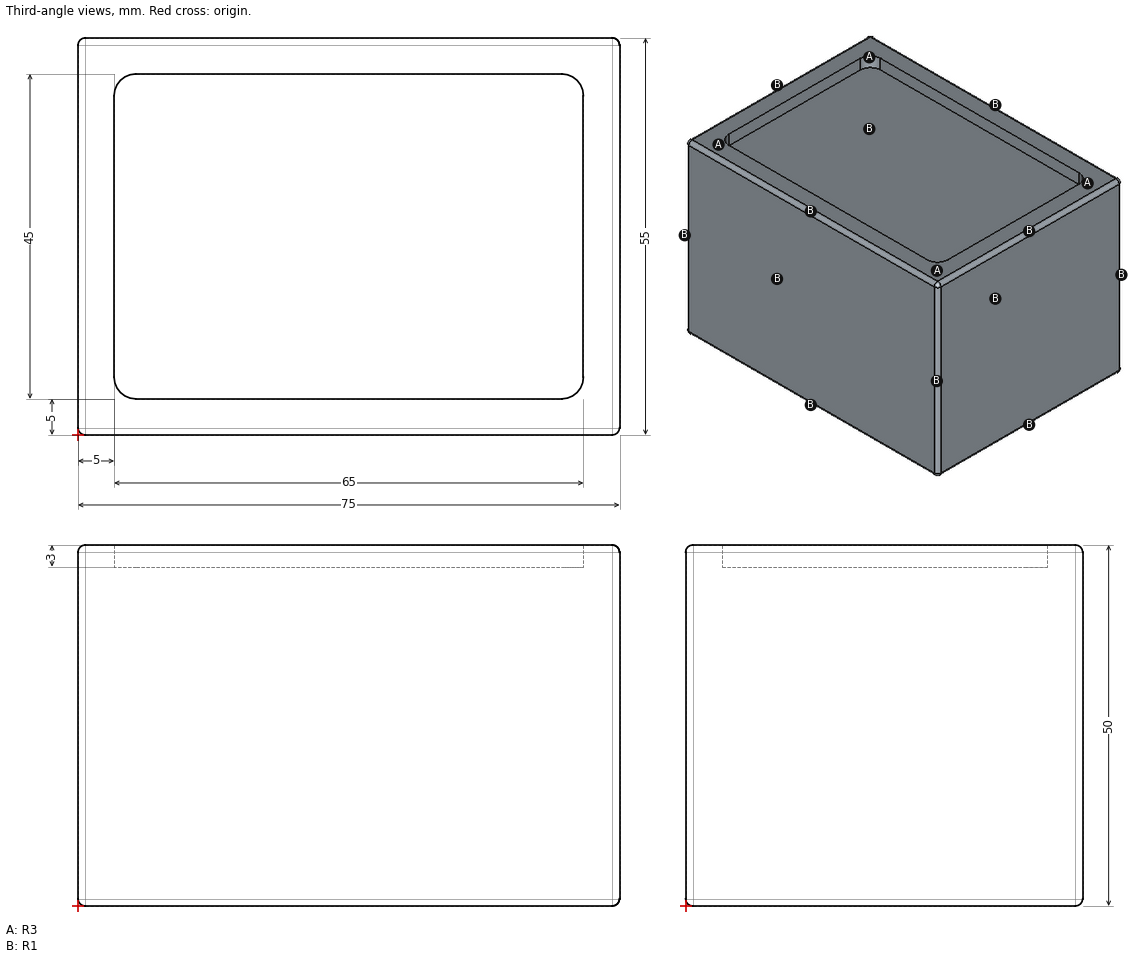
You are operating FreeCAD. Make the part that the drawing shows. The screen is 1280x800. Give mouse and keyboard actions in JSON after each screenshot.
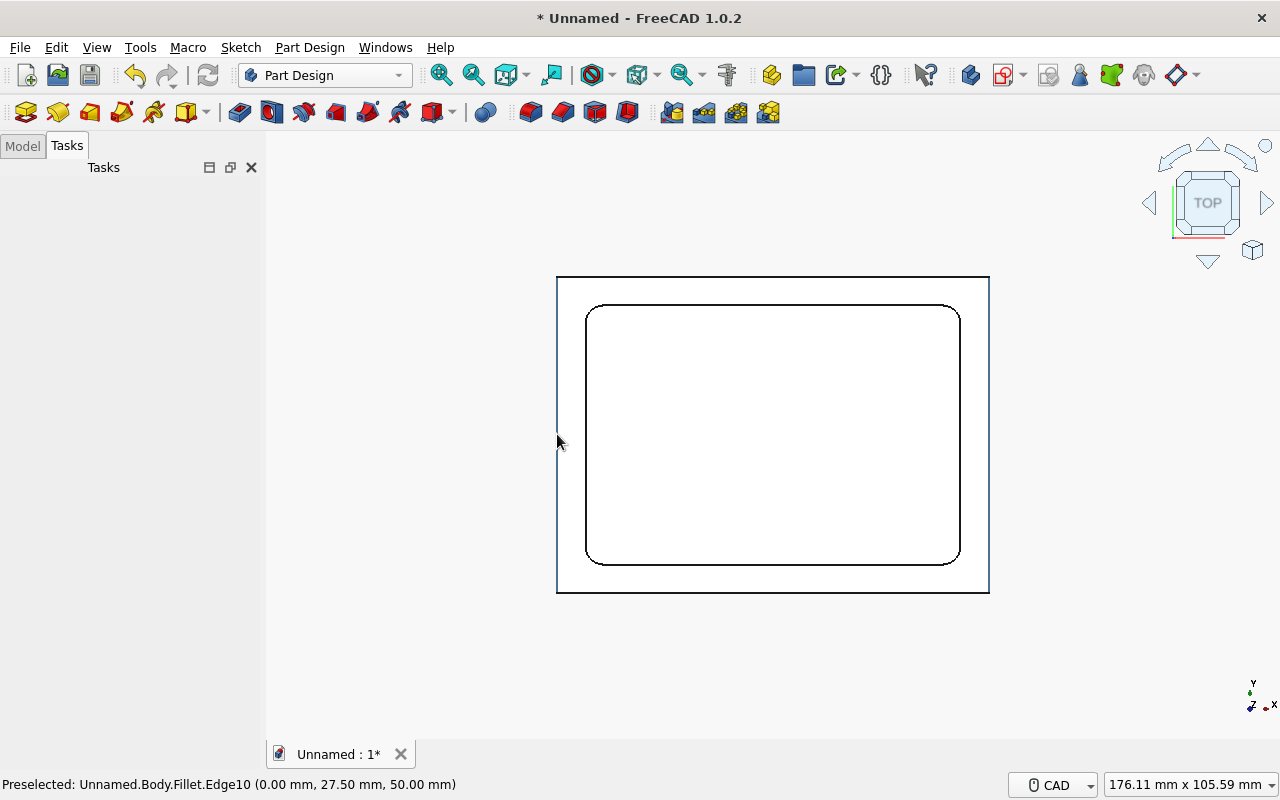
{"action": "key", "text": "0"}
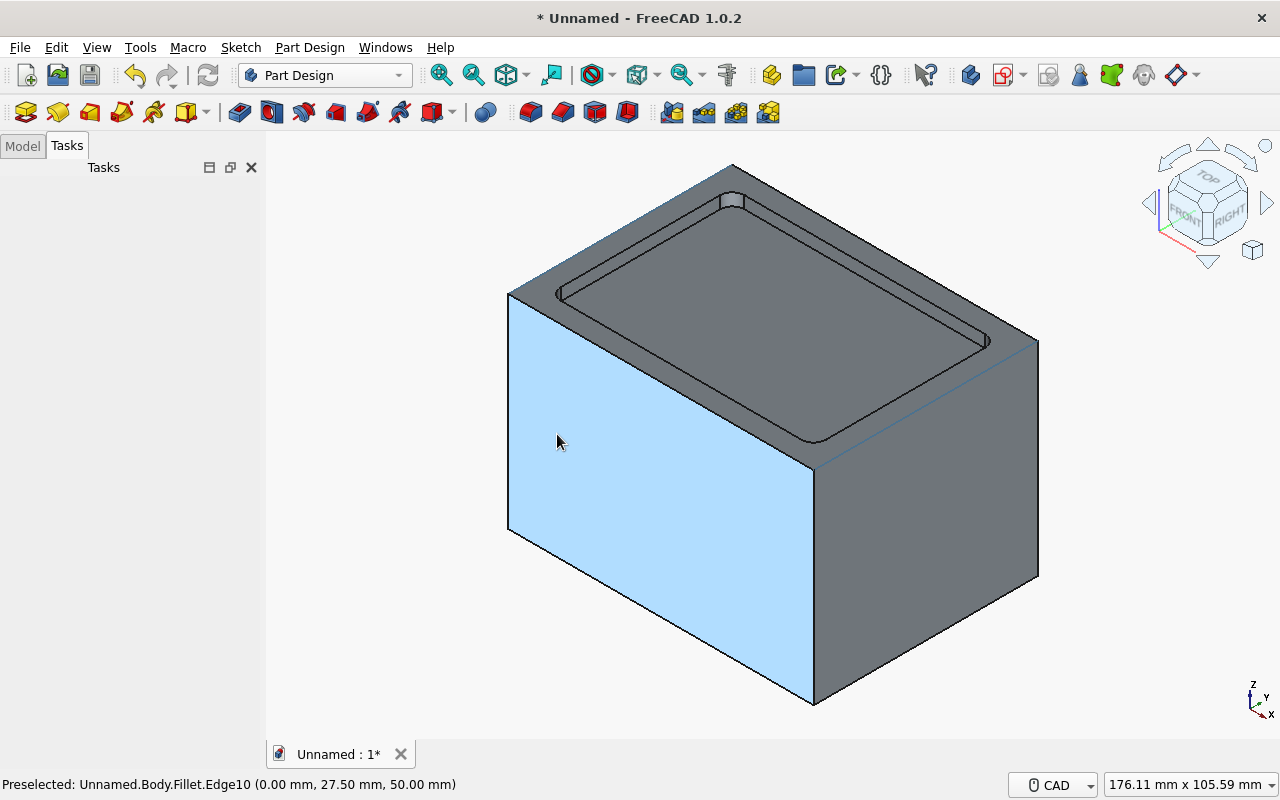
{"action": "key", "text": "1"}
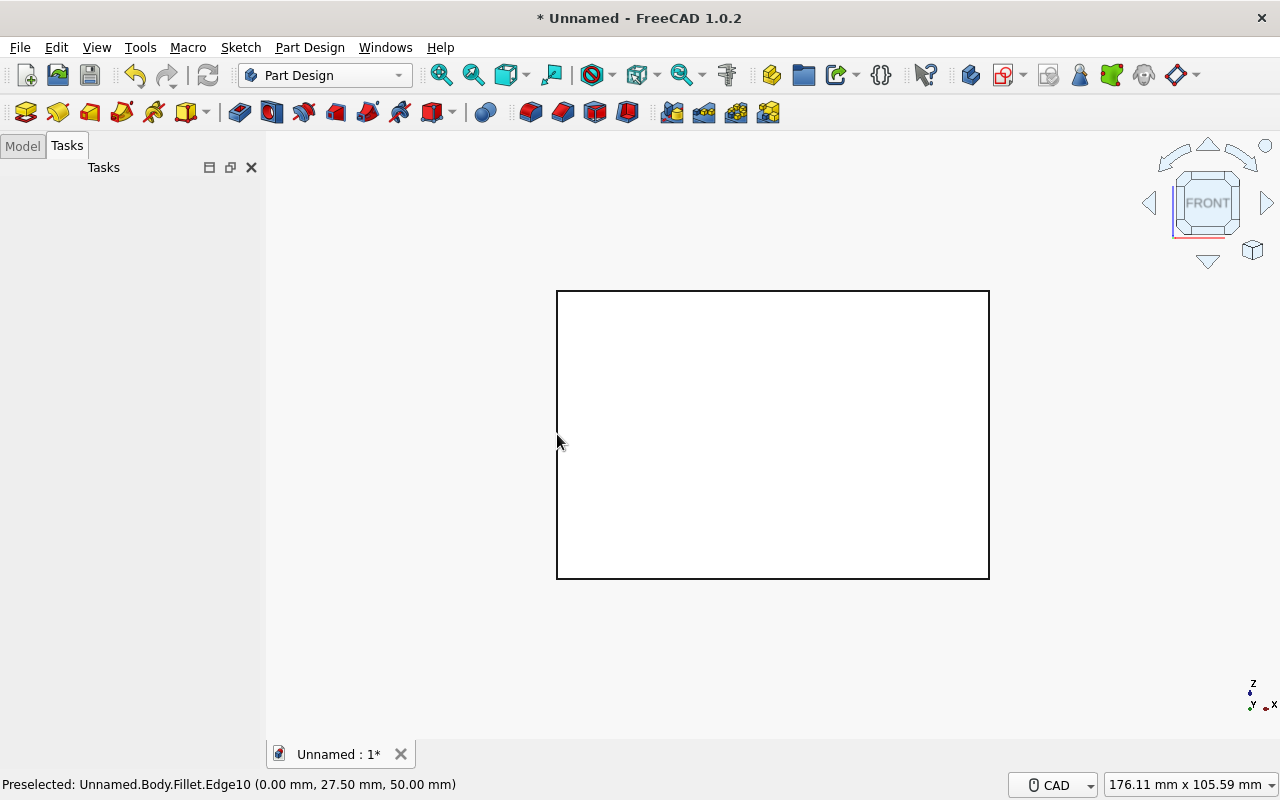
{"action": "key", "text": "3"}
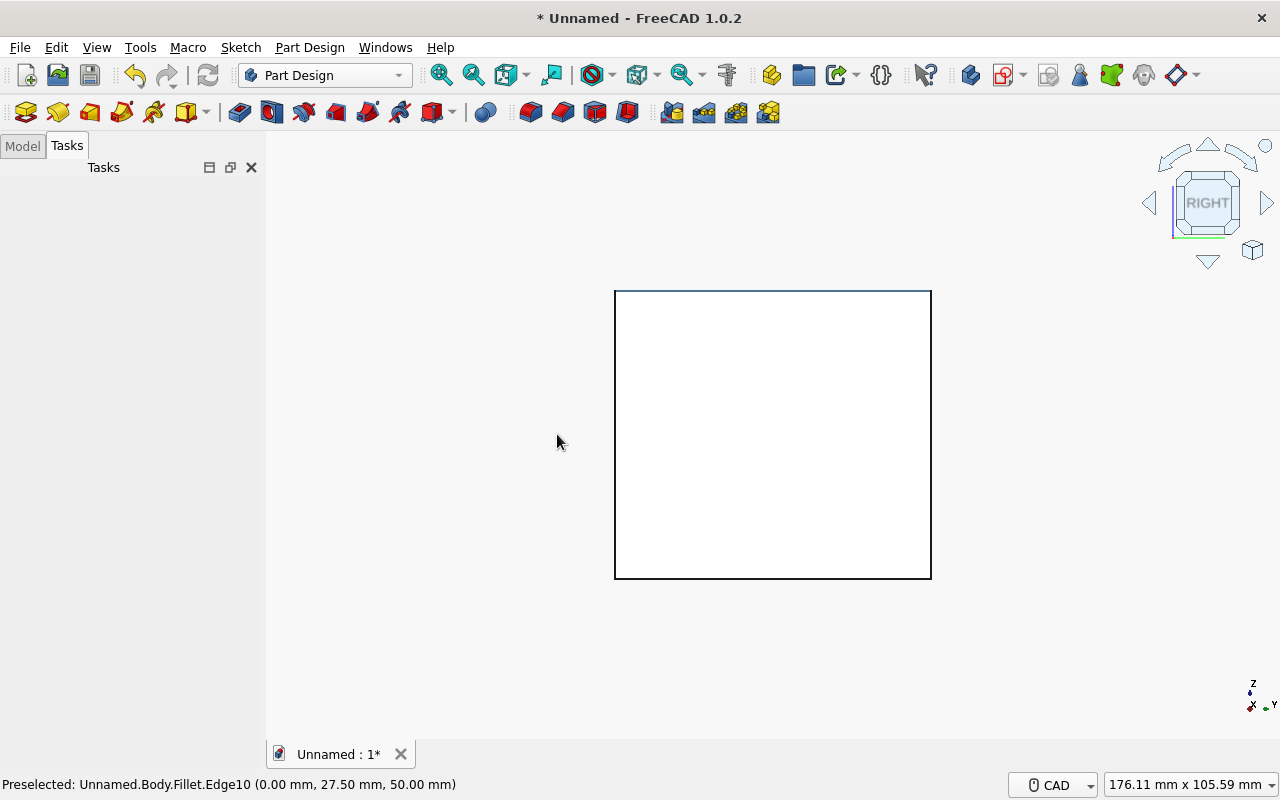
{"action": "key", "text": "5"}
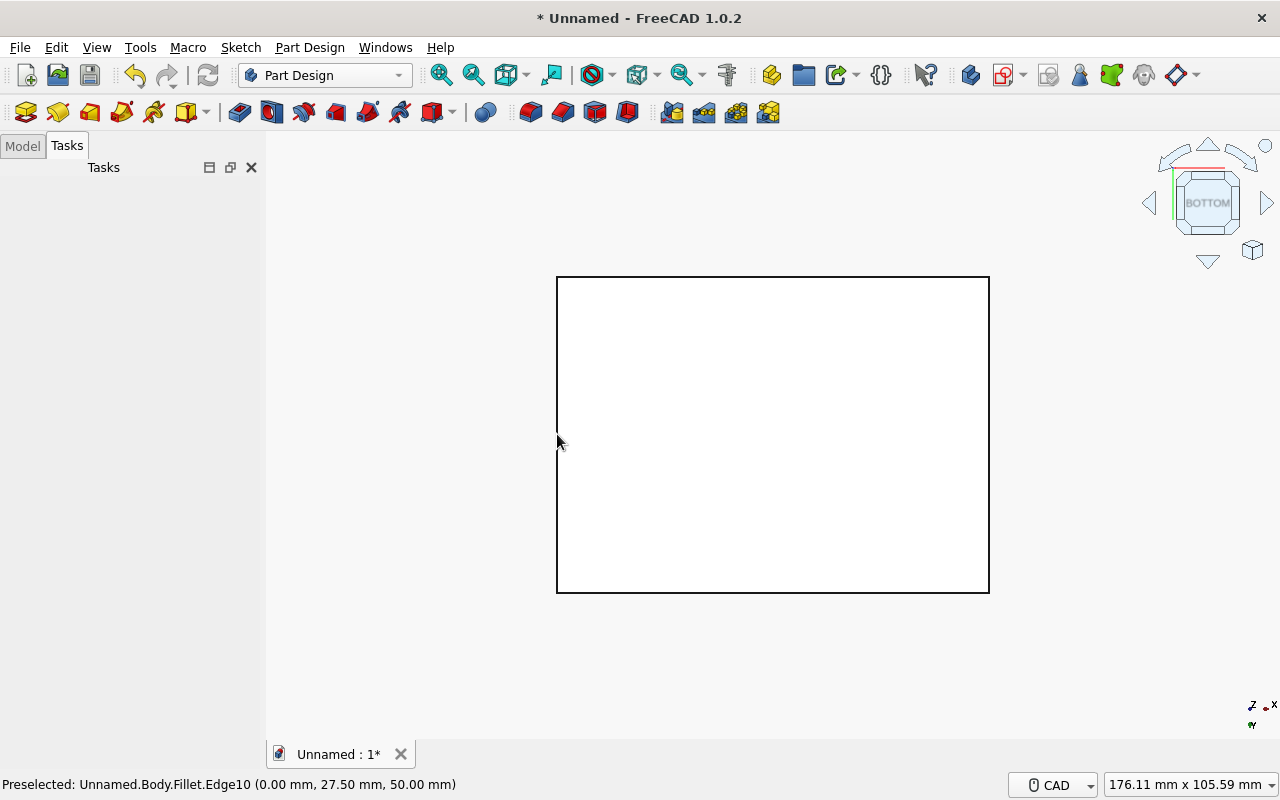
{"action": "left_click", "coordinate": [773, 434], "text": "ctrl"}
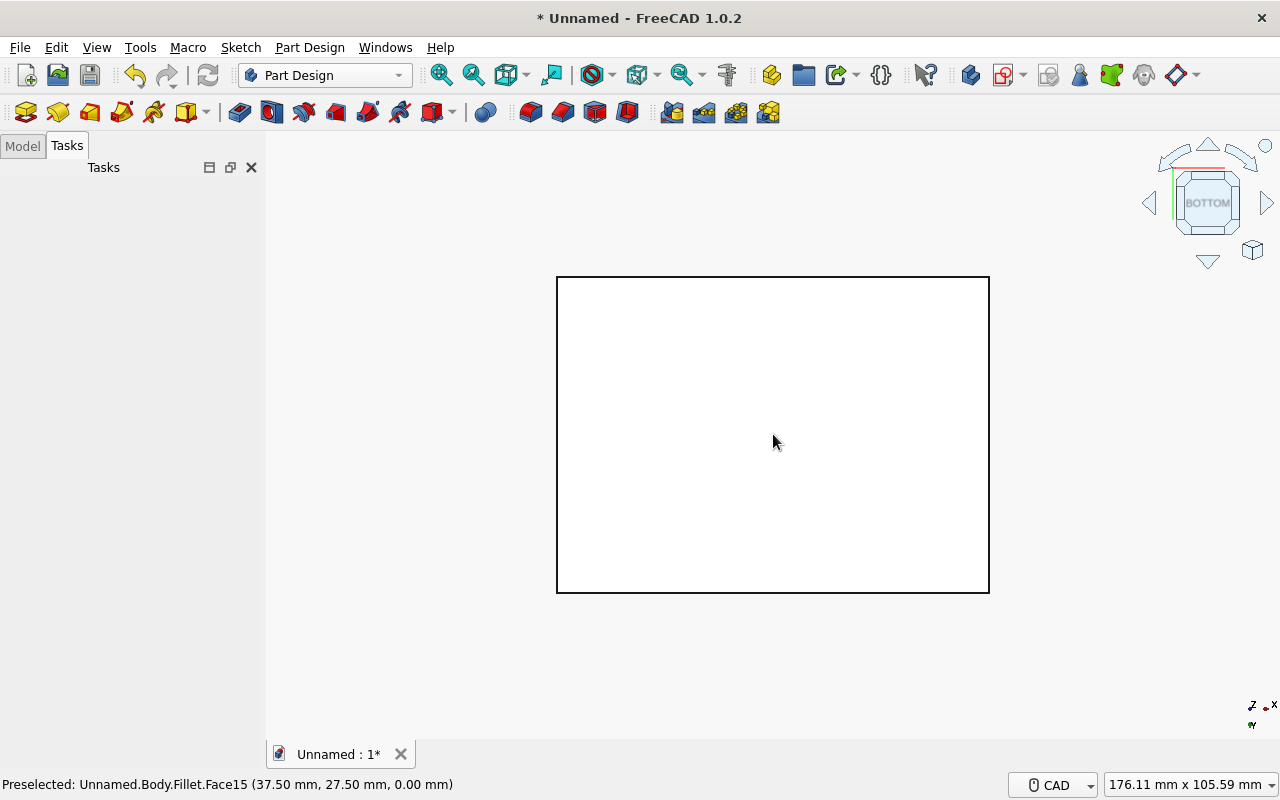
{"action": "key", "text": "4"}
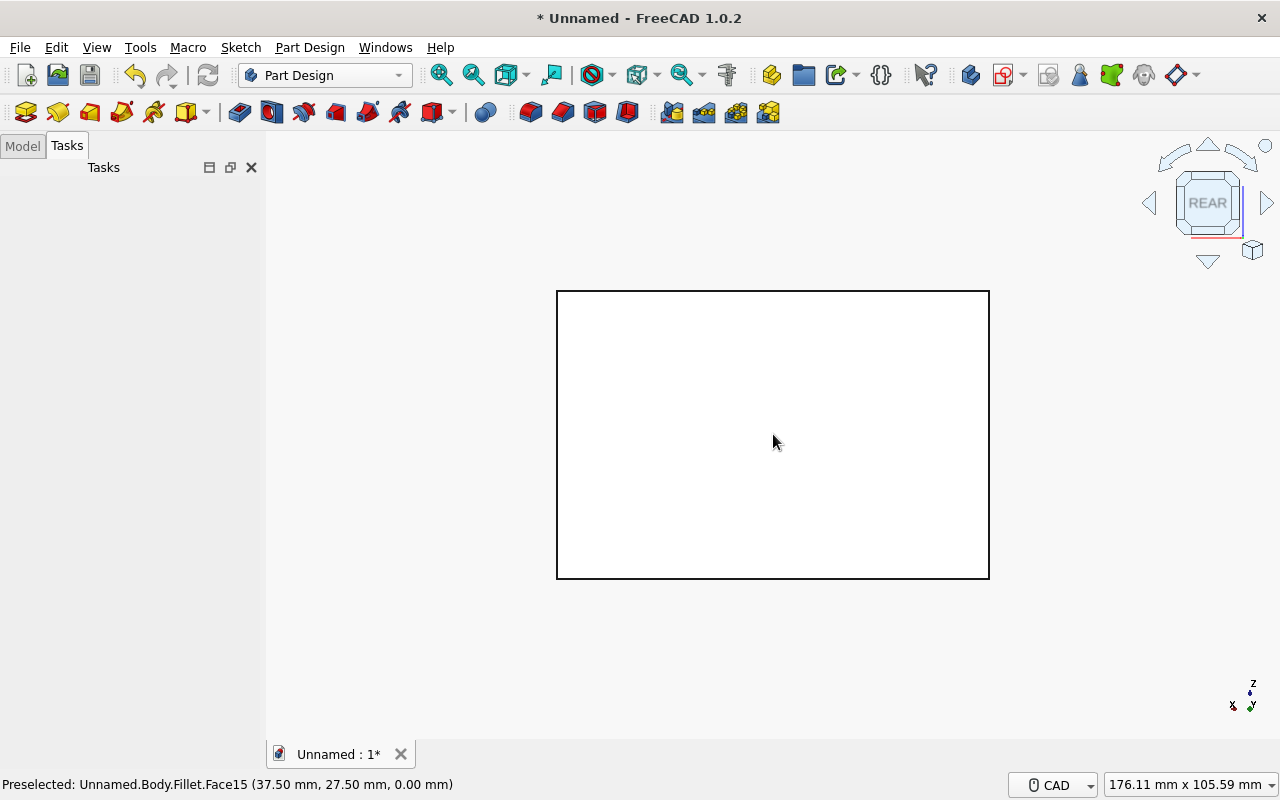
{"action": "left_click", "coordinate": [711, 434], "text": "ctrl"}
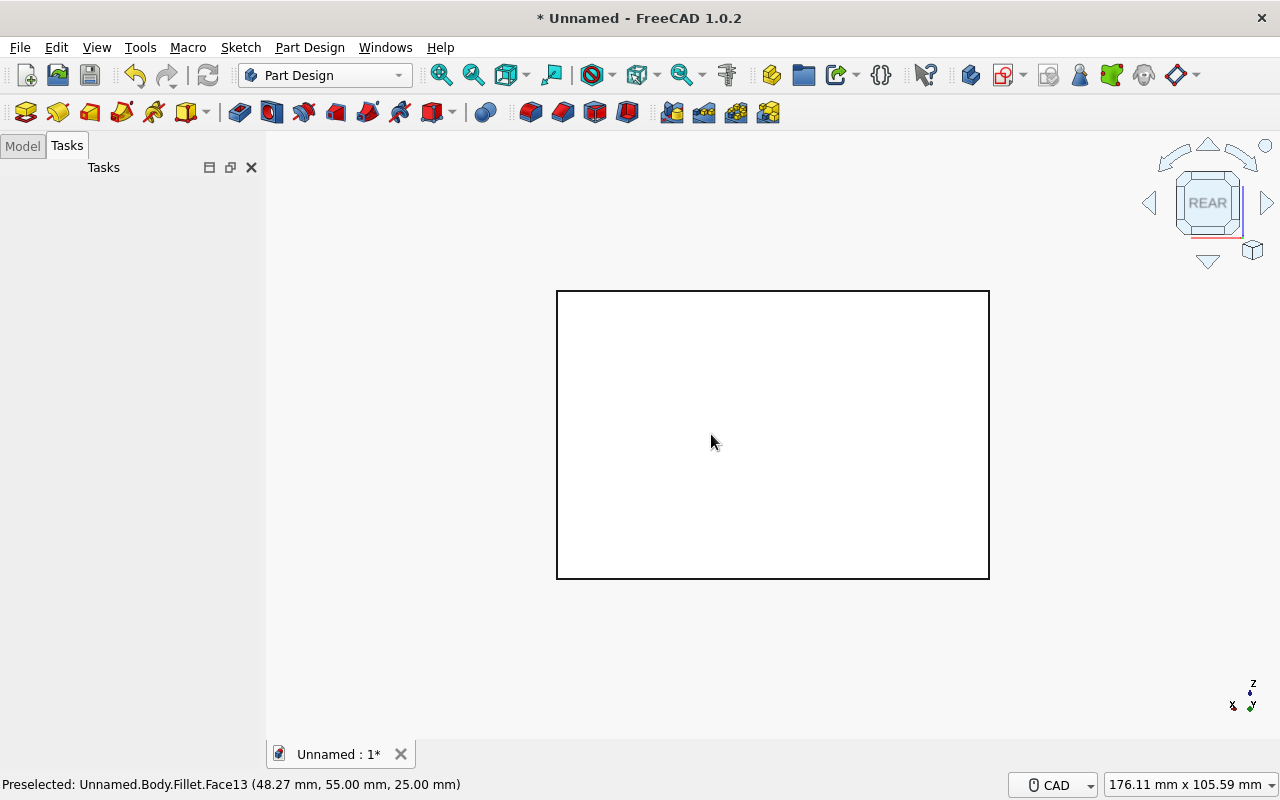
{"action": "left_click", "coordinate": [532, 112]}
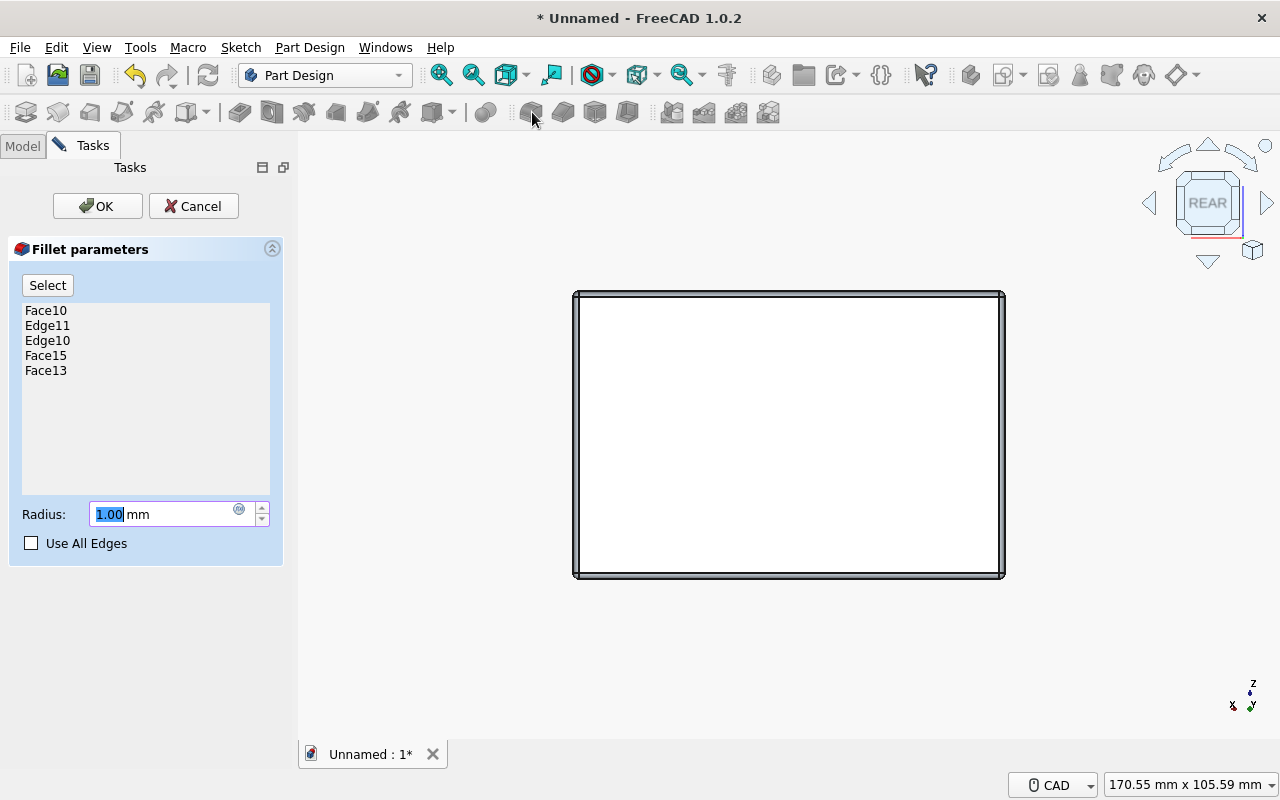
{"action": "type", "text": "1"}
{"action": "key", "text": "Tab"}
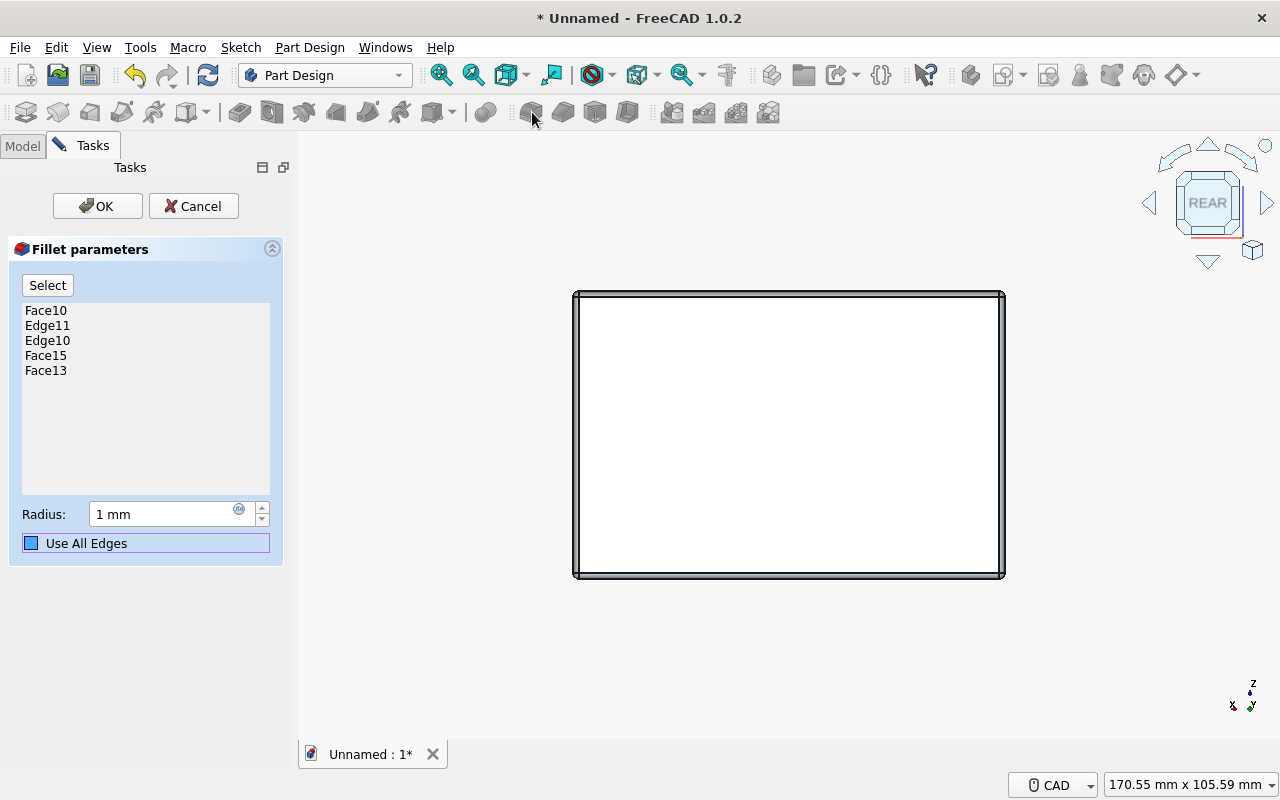
{"action": "left_click", "coordinate": [98, 206]}